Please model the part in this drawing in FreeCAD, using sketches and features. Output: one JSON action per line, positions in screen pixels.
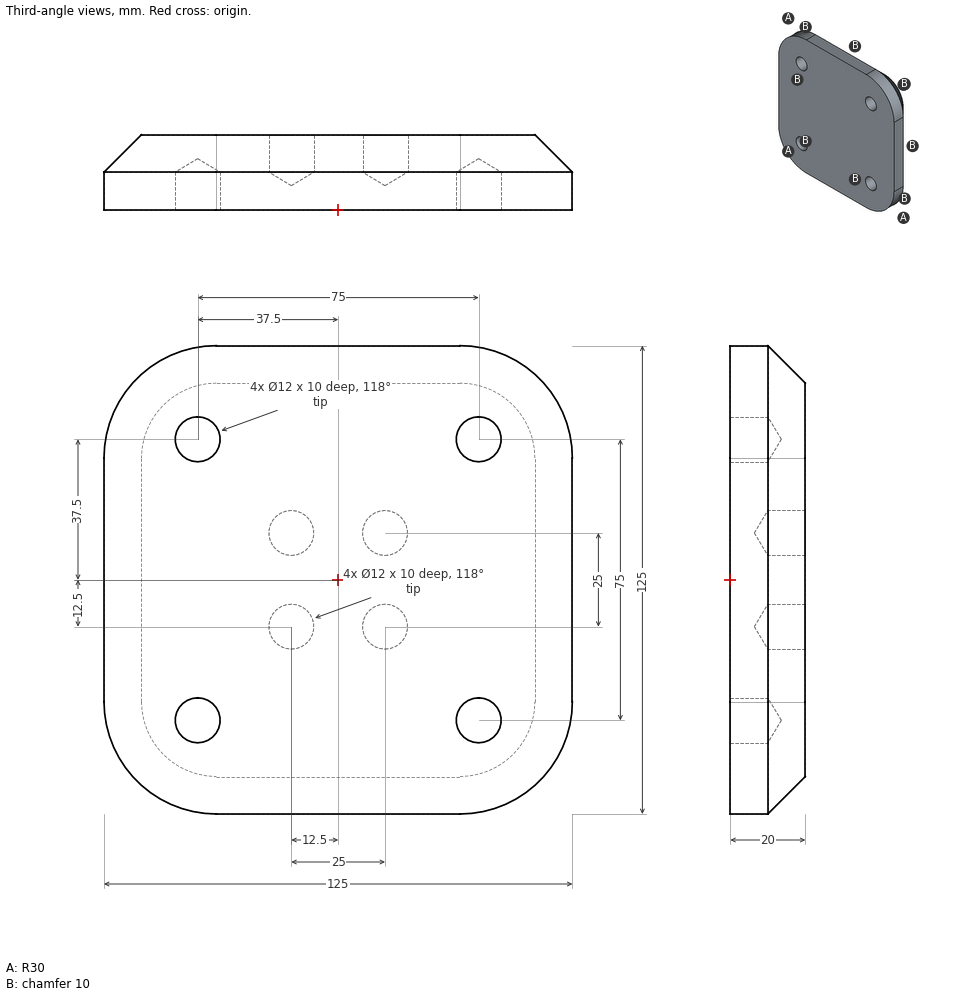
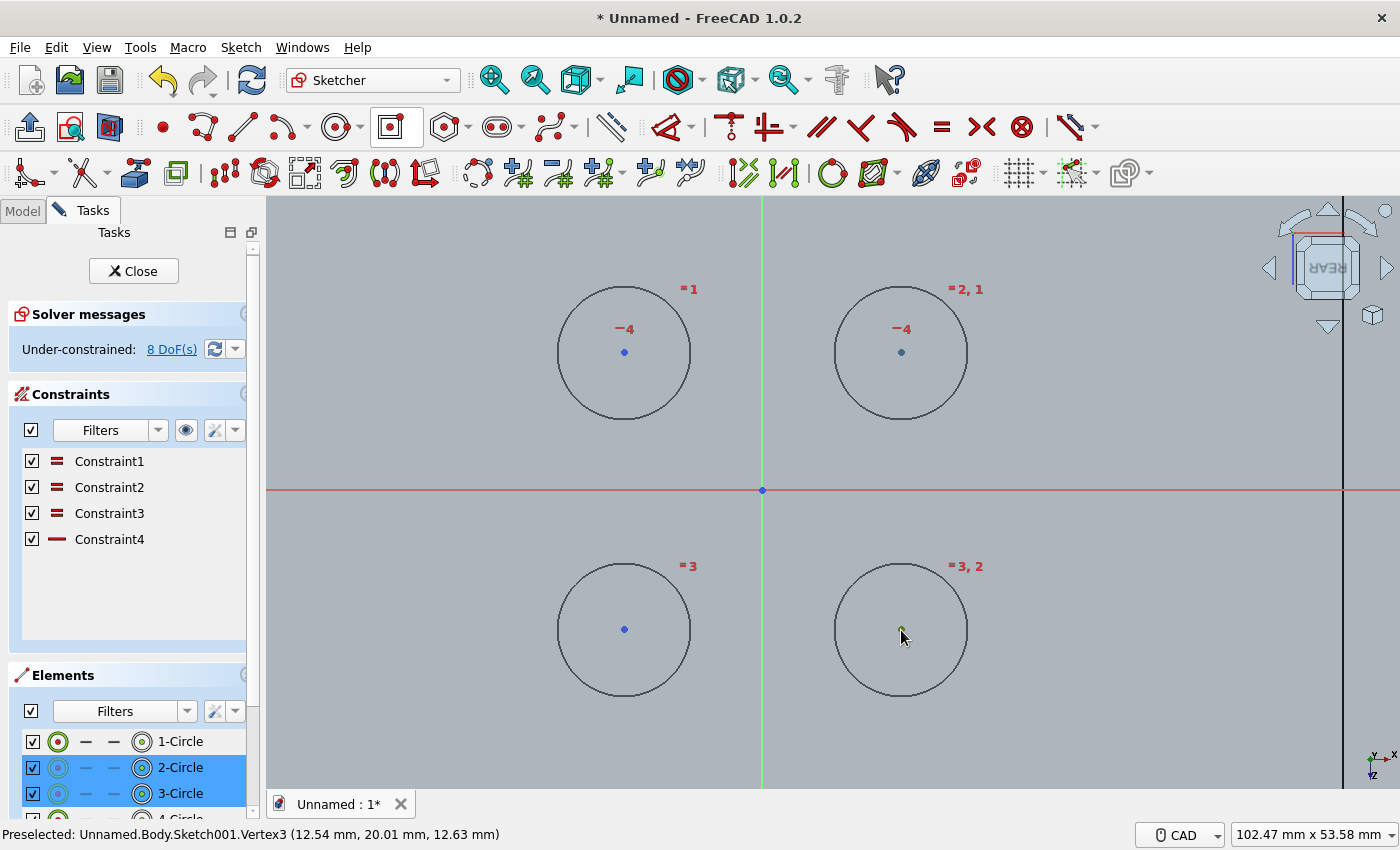
{"action": "key", "text": "v"}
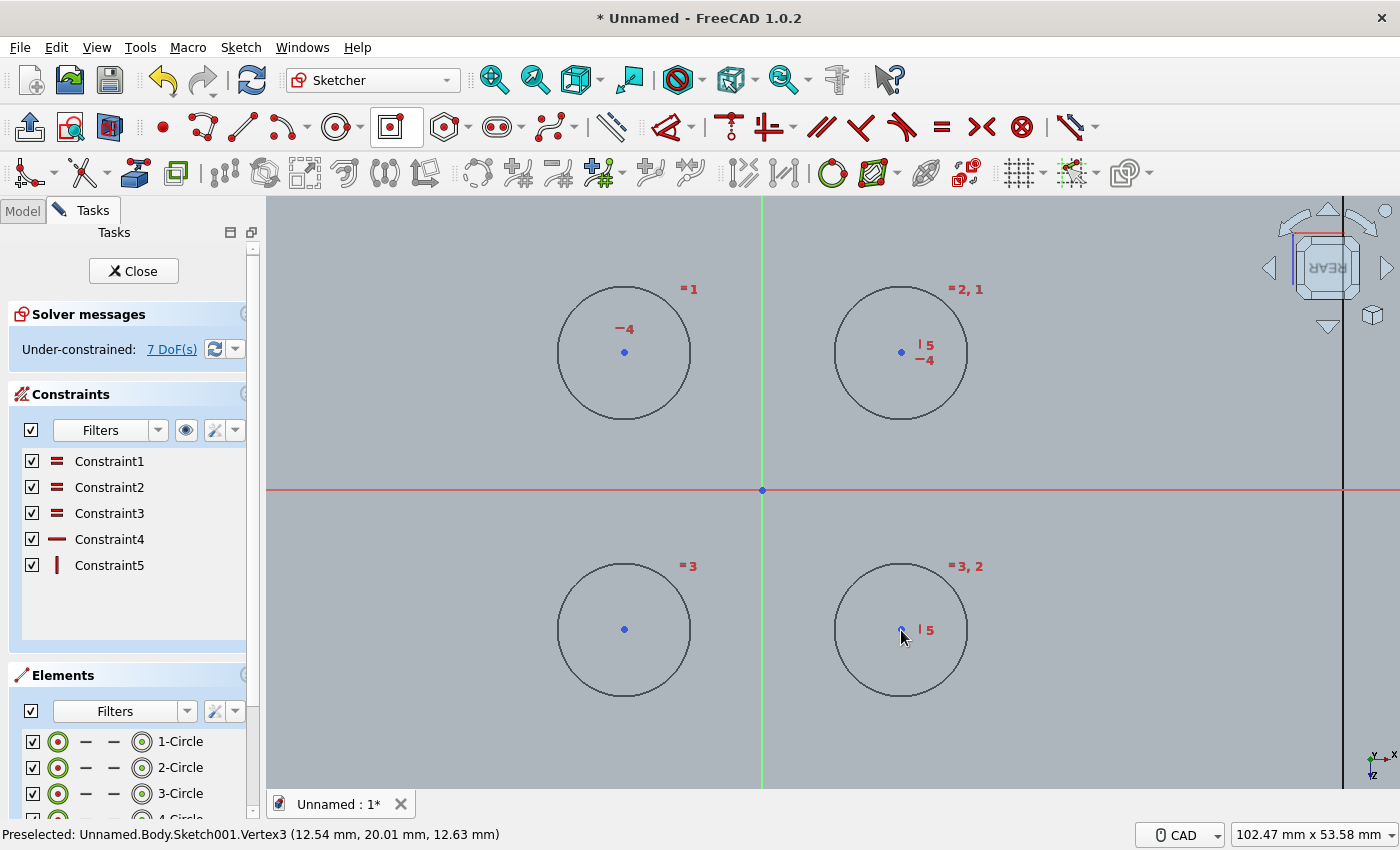
{"action": "left_click", "coordinate": [624, 353]}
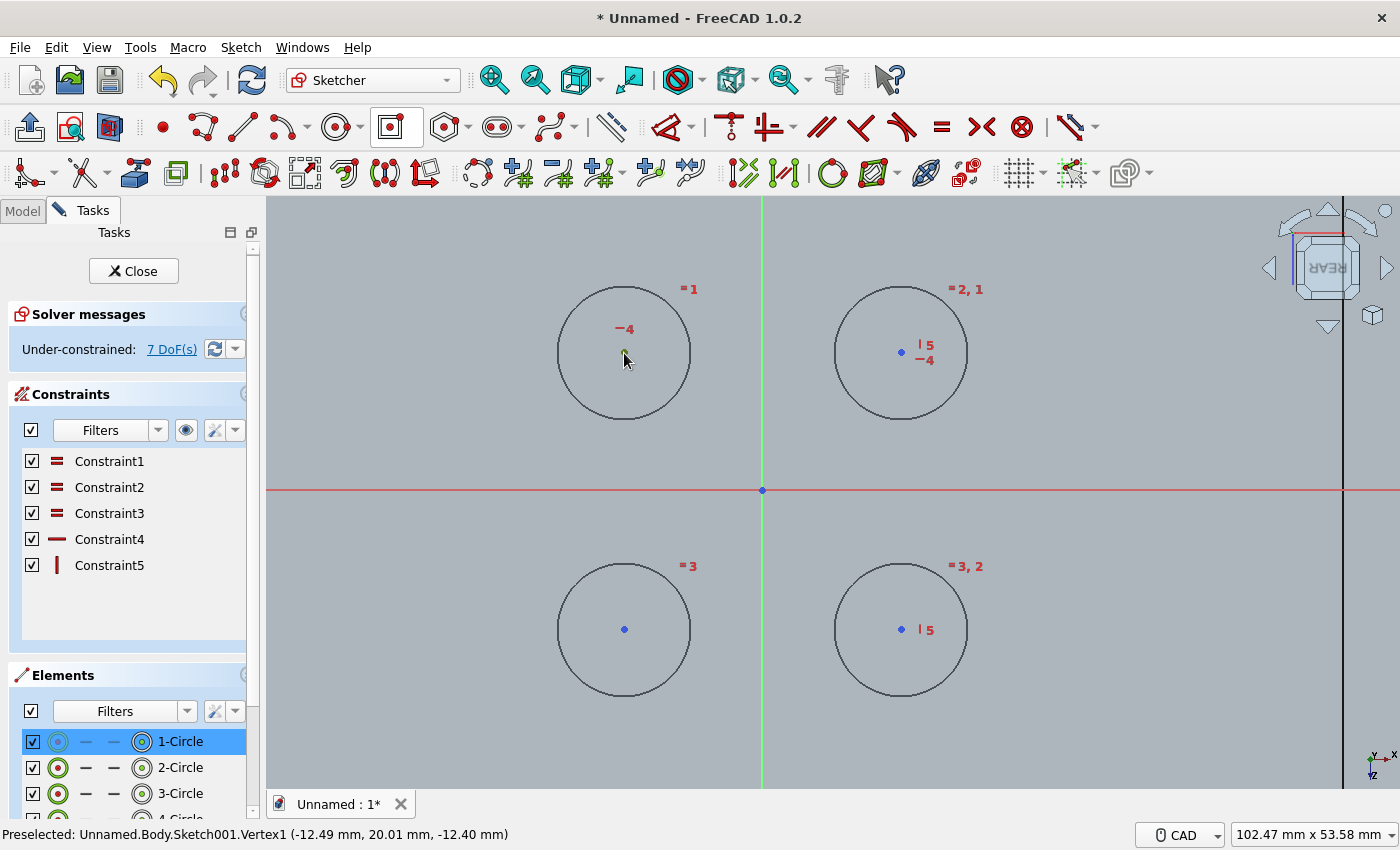
{"action": "left_click", "coordinate": [624, 630]}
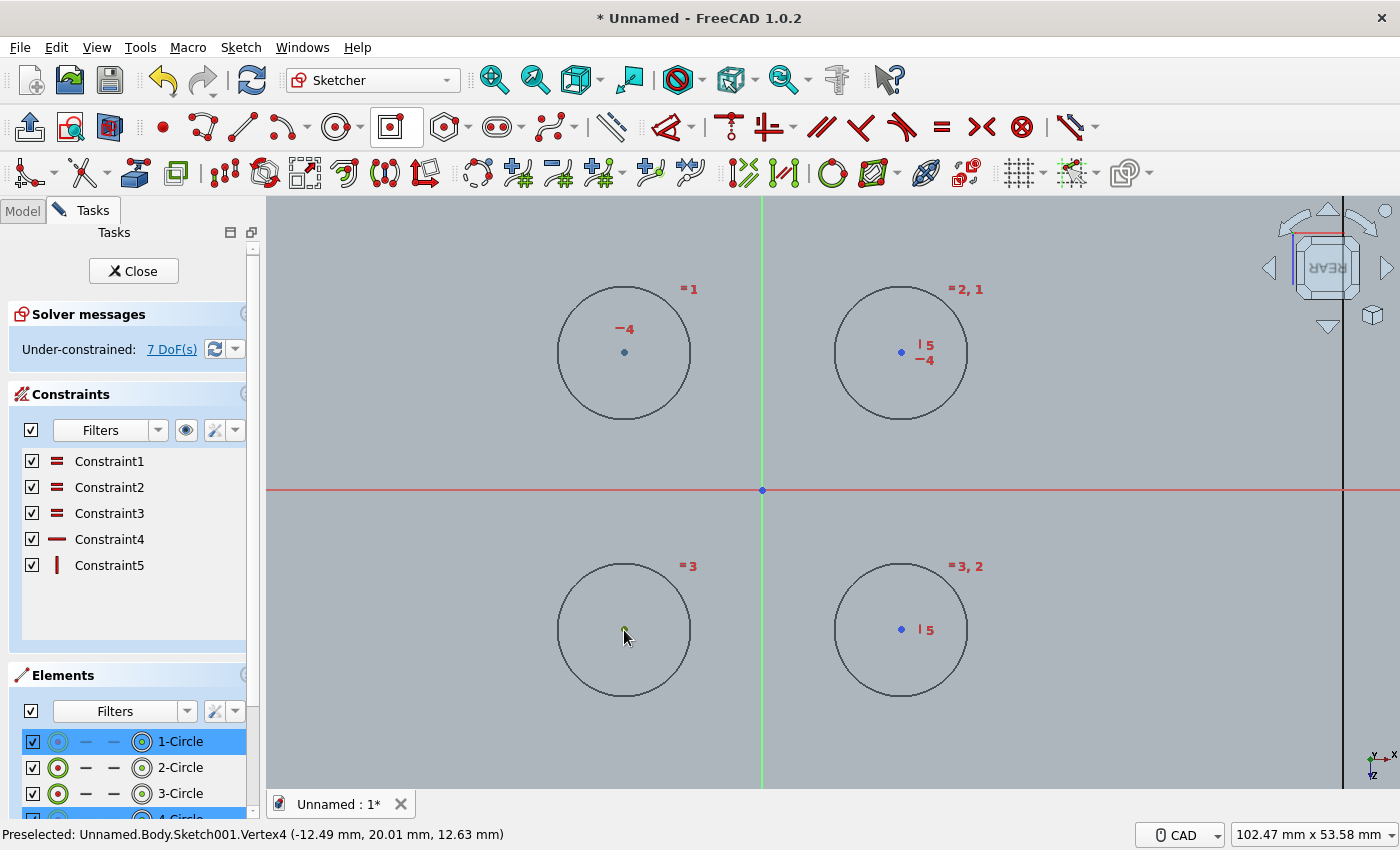
{"action": "key", "text": "v"}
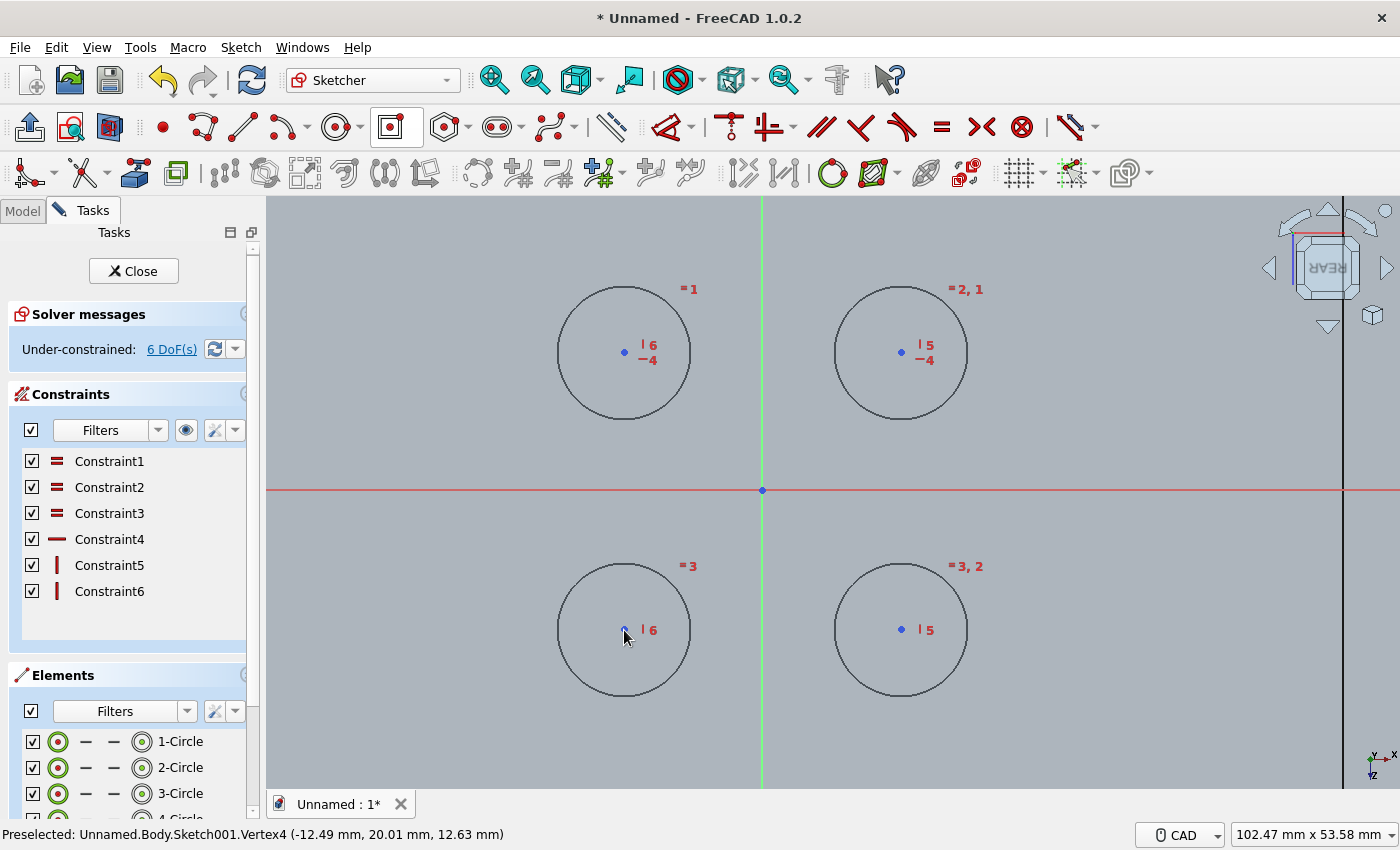
{"action": "left_click", "coordinate": [901, 630]}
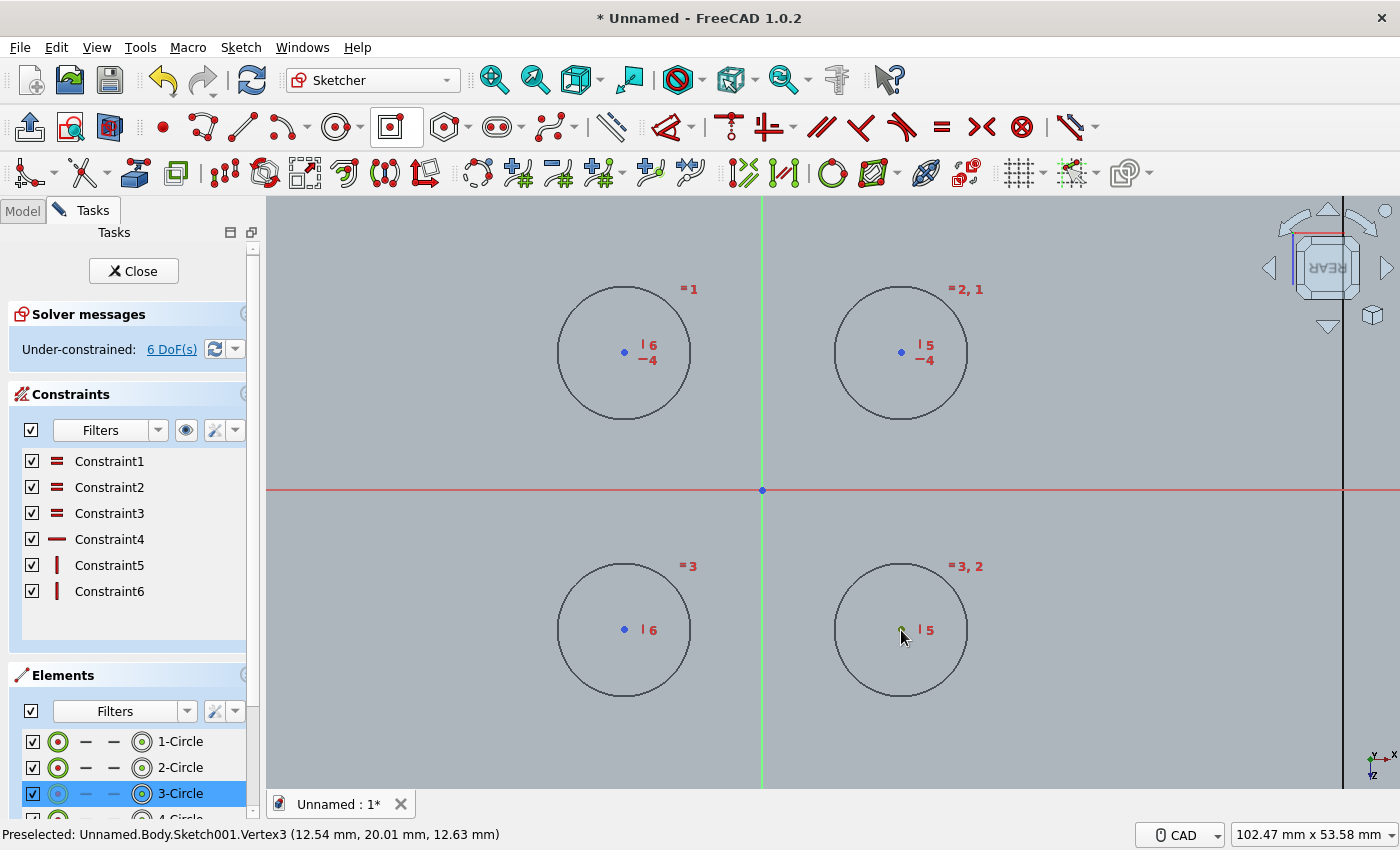
{"action": "left_click", "coordinate": [624, 630]}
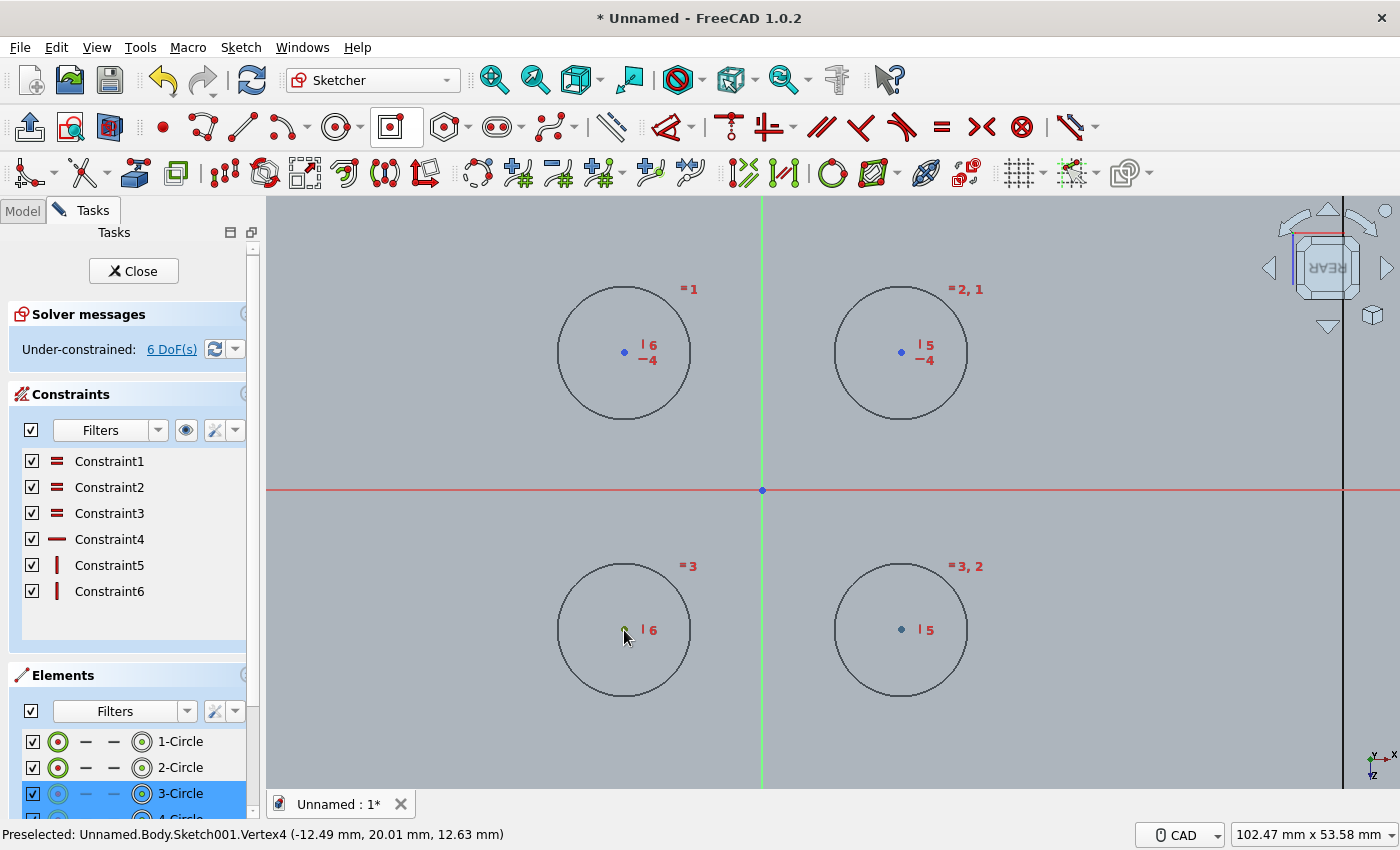
{"action": "left_click", "coordinate": [796, 128]}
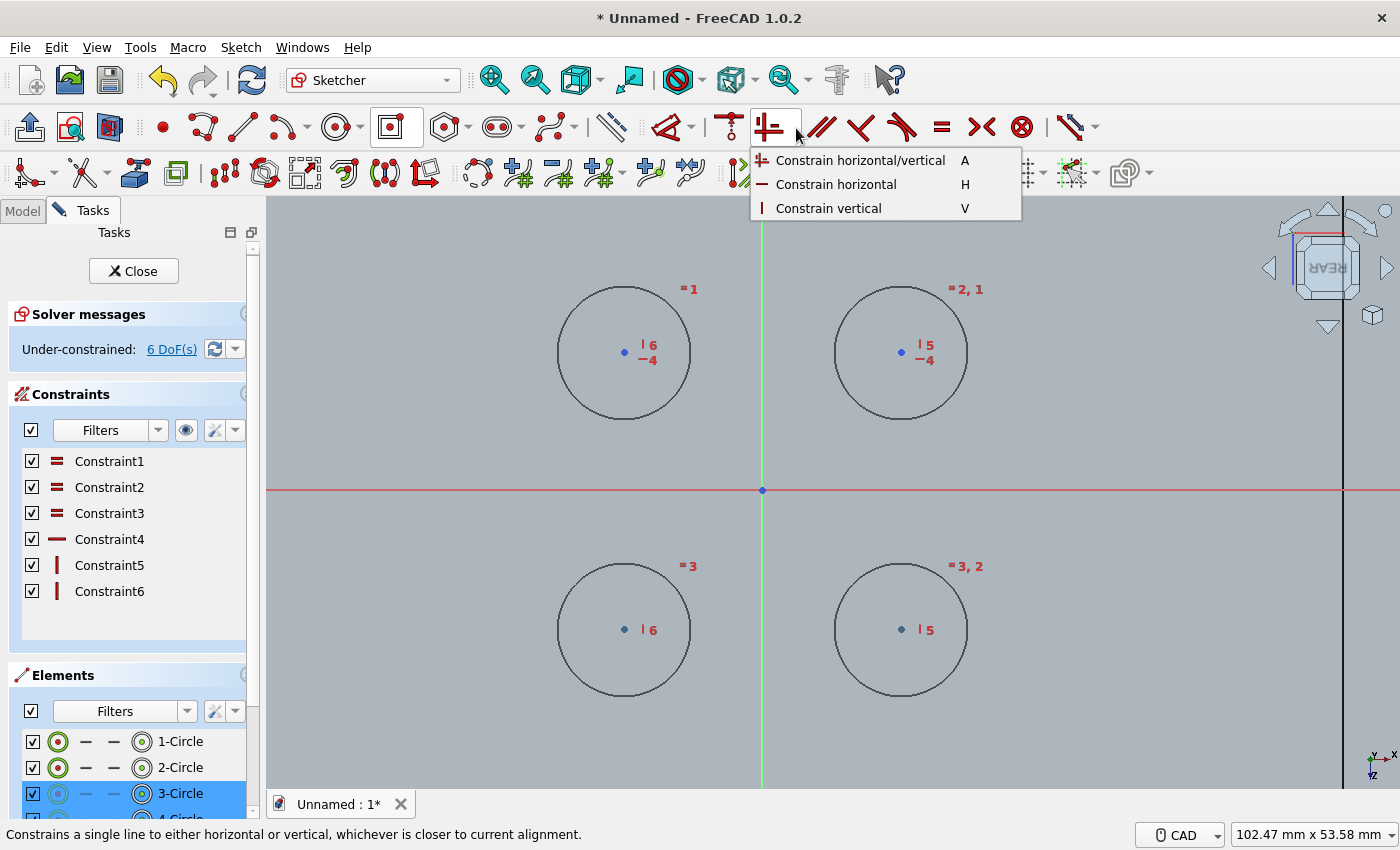
{"action": "left_click", "coordinate": [886, 184]}